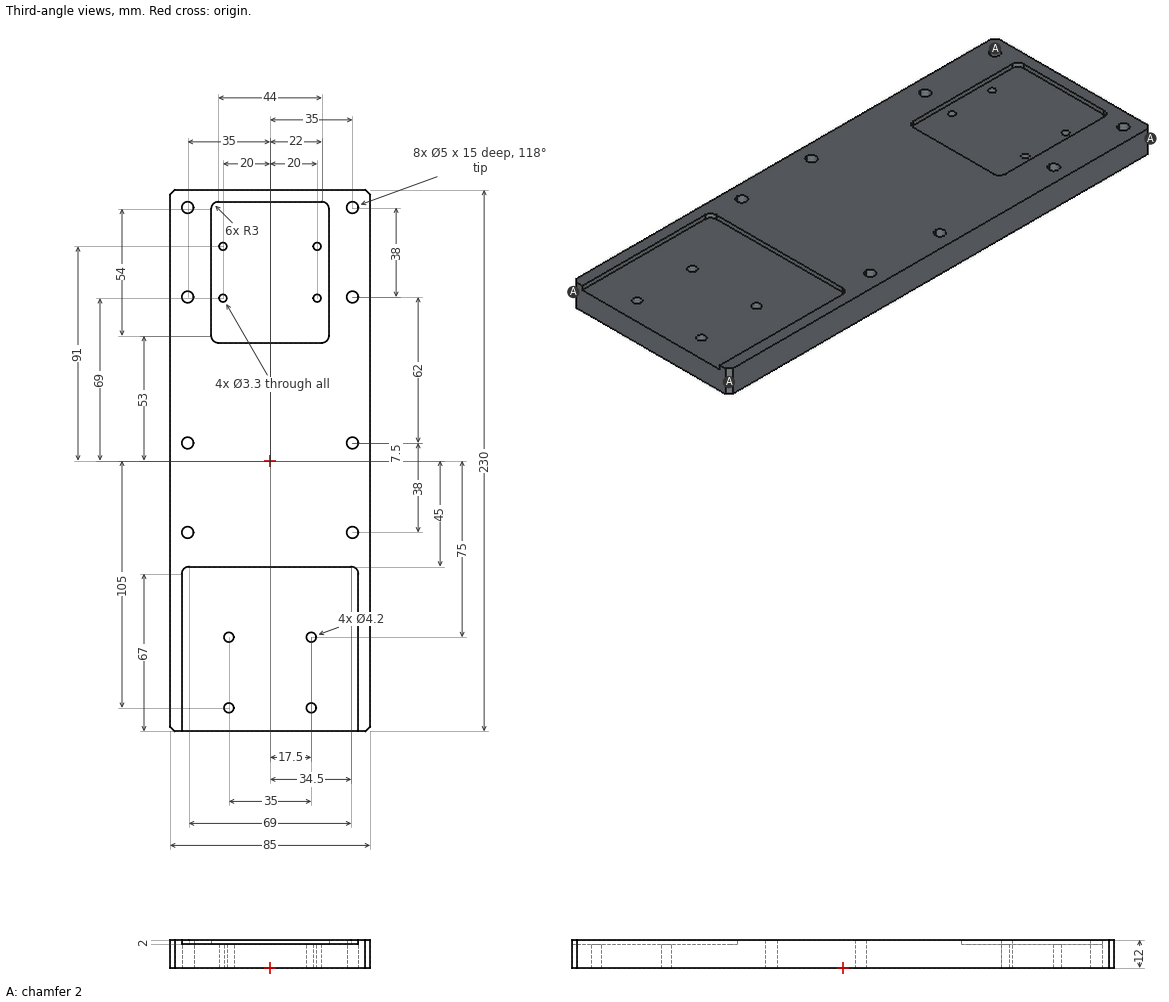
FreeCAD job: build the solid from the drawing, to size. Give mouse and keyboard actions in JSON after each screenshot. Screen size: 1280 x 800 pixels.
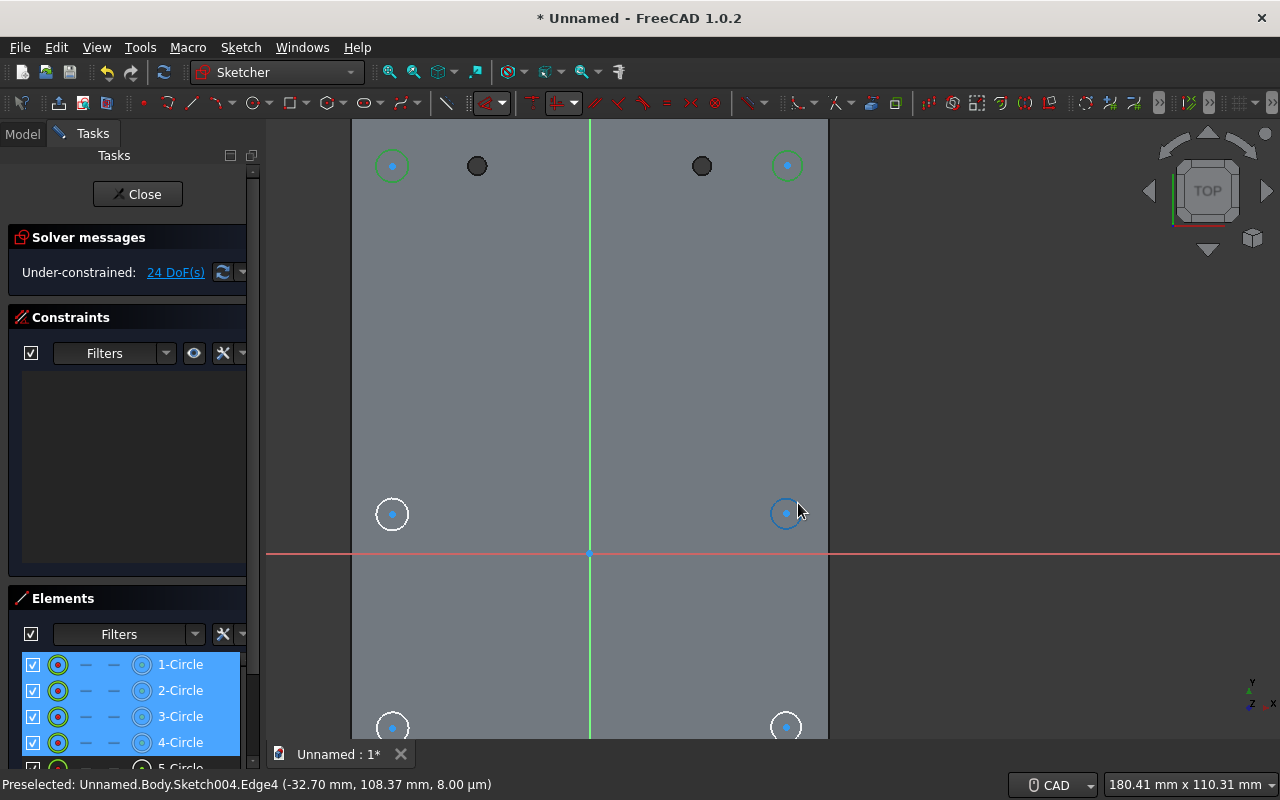
{"action": "left_click", "coordinate": [797, 503]}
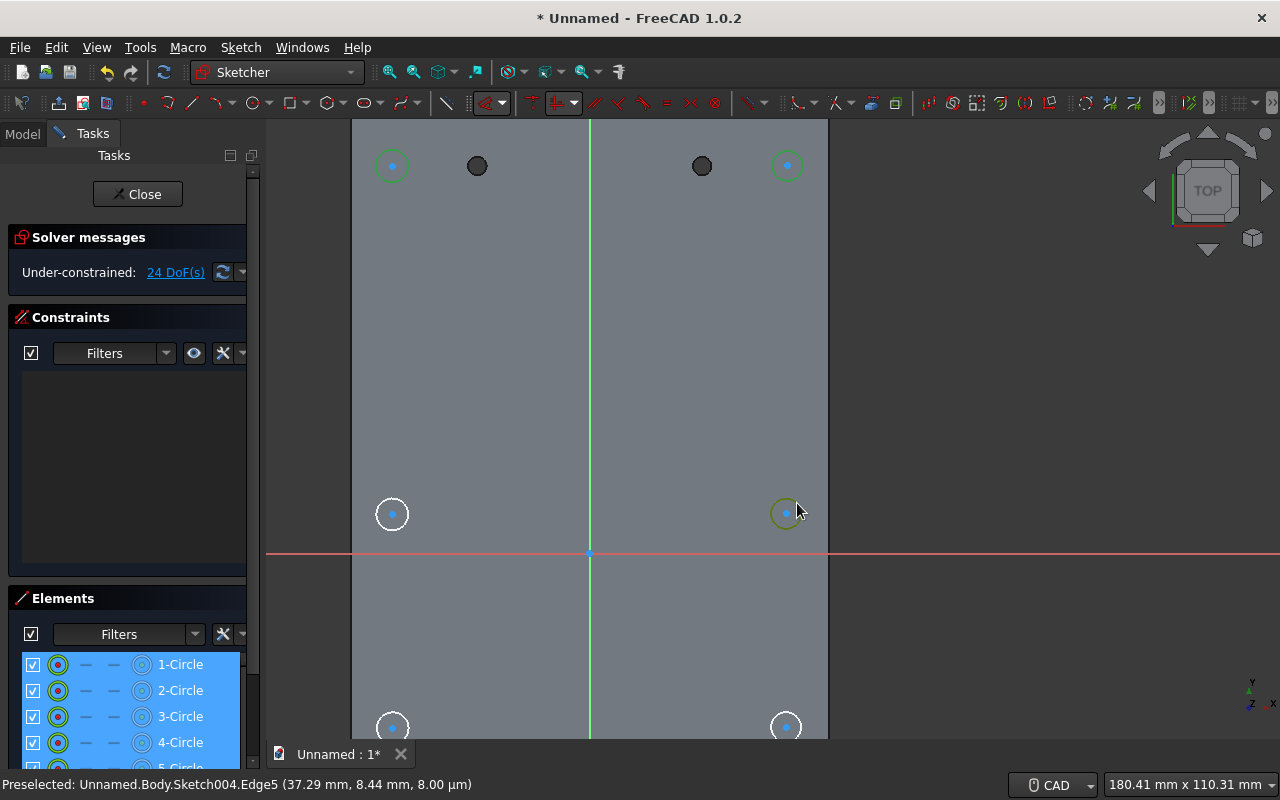
{"action": "scroll", "coordinate": [798, 504], "scroll_direction": "down", "scroll_amount": 4}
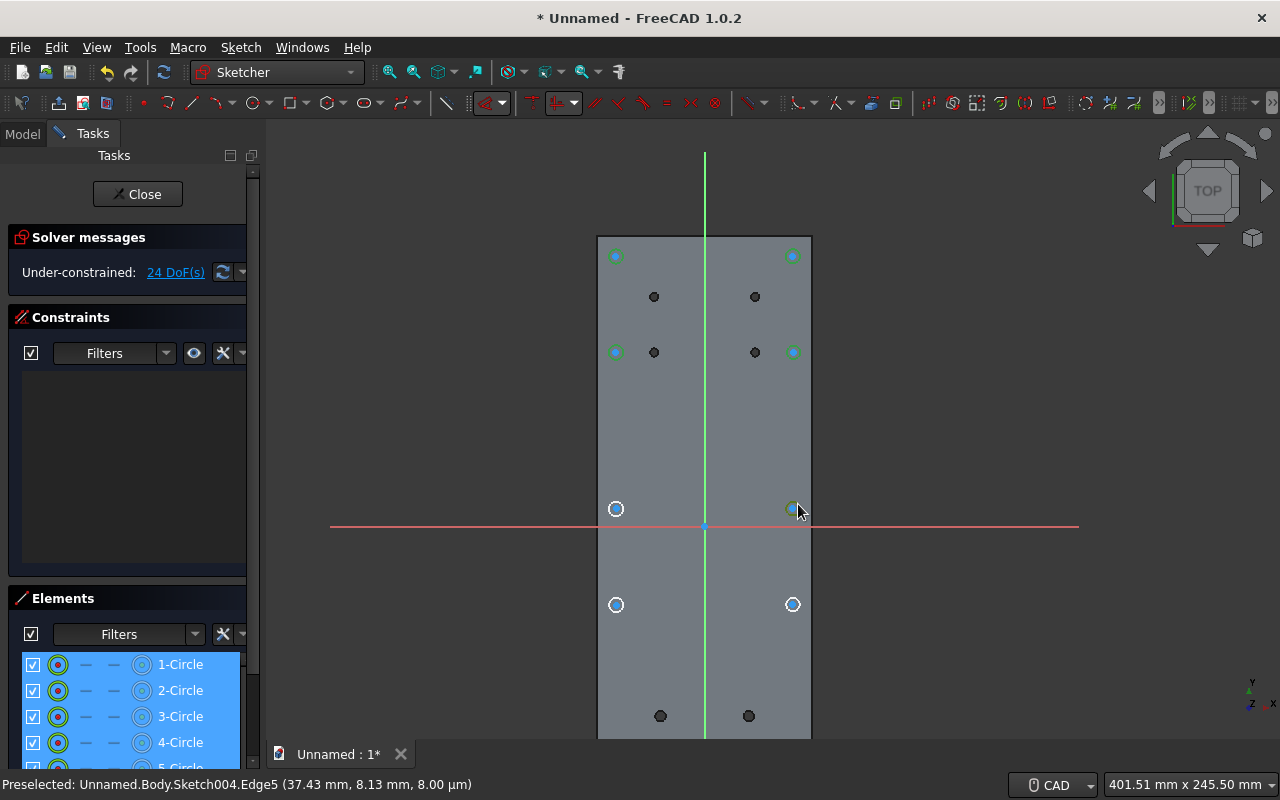
{"action": "scroll", "coordinate": [798, 600], "scroll_direction": "up", "scroll_amount": 4}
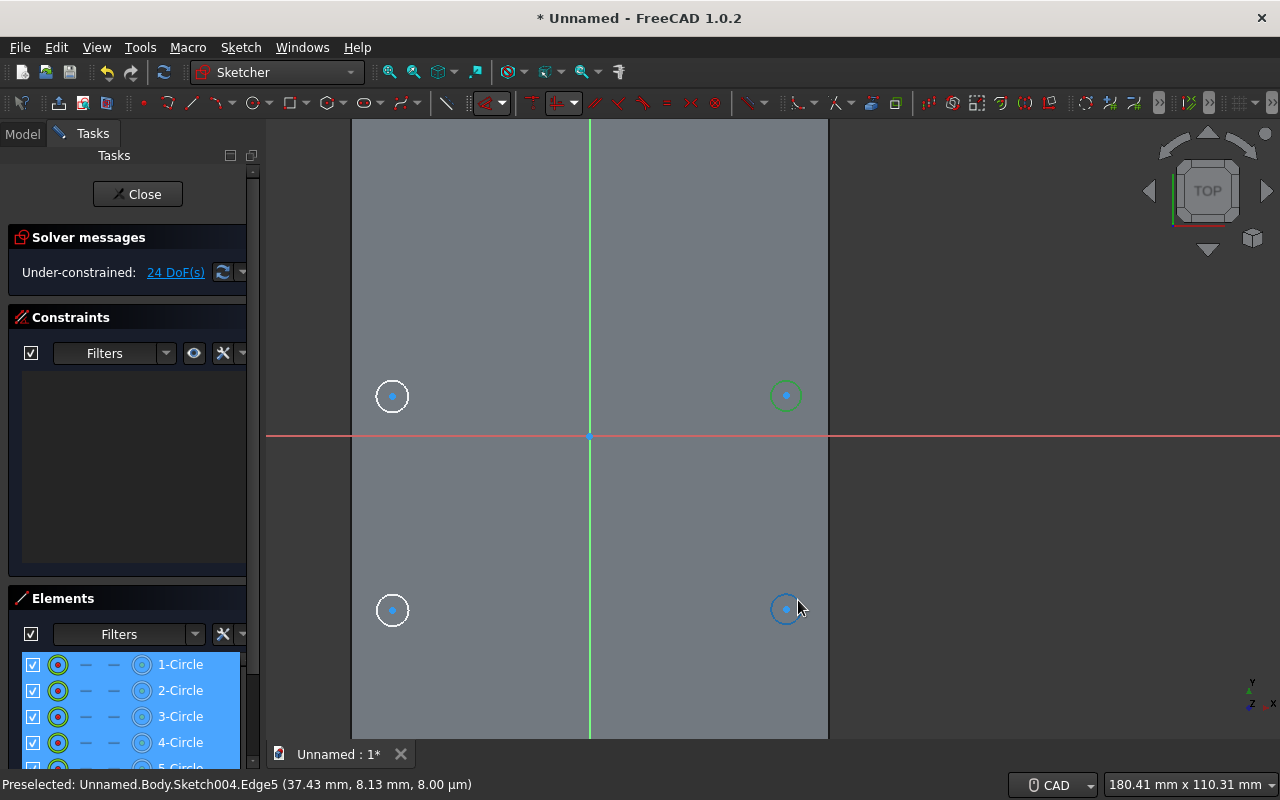
{"action": "left_click", "coordinate": [797, 599]}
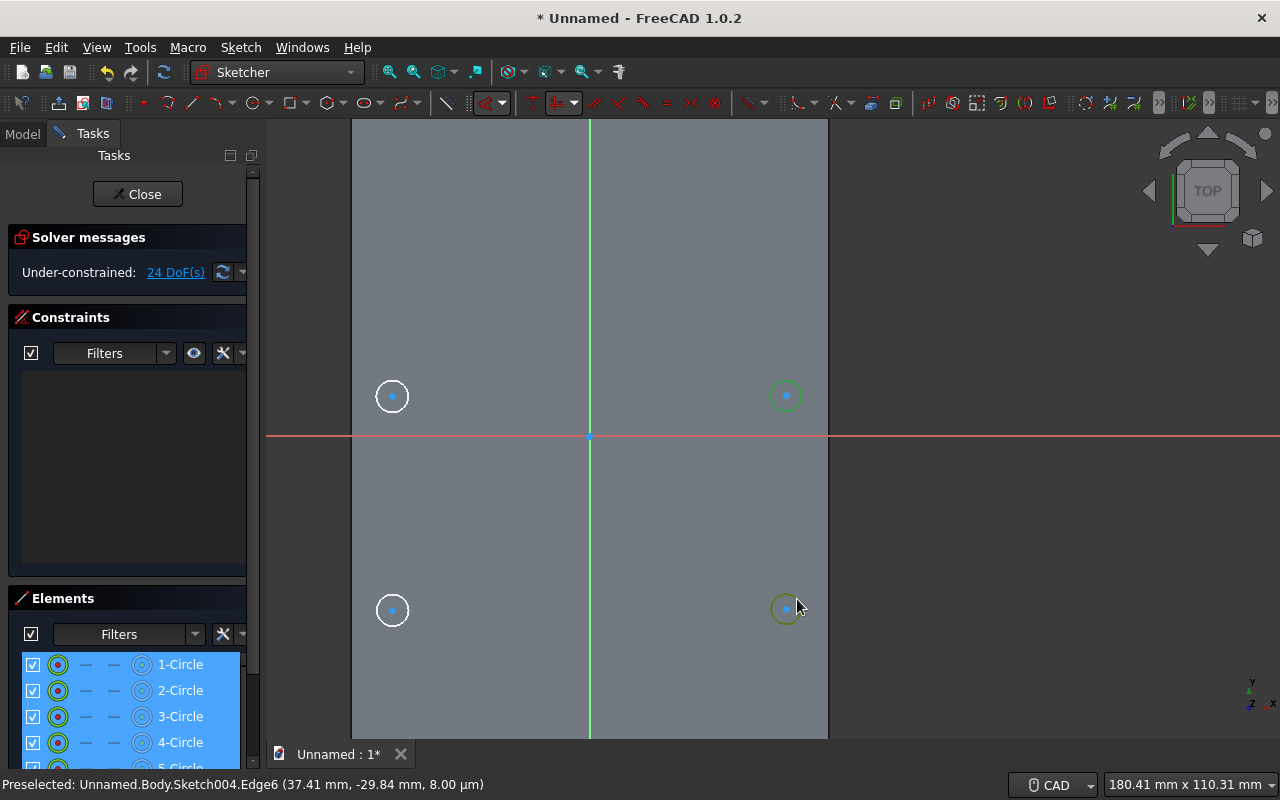
{"action": "left_click", "coordinate": [404, 599]}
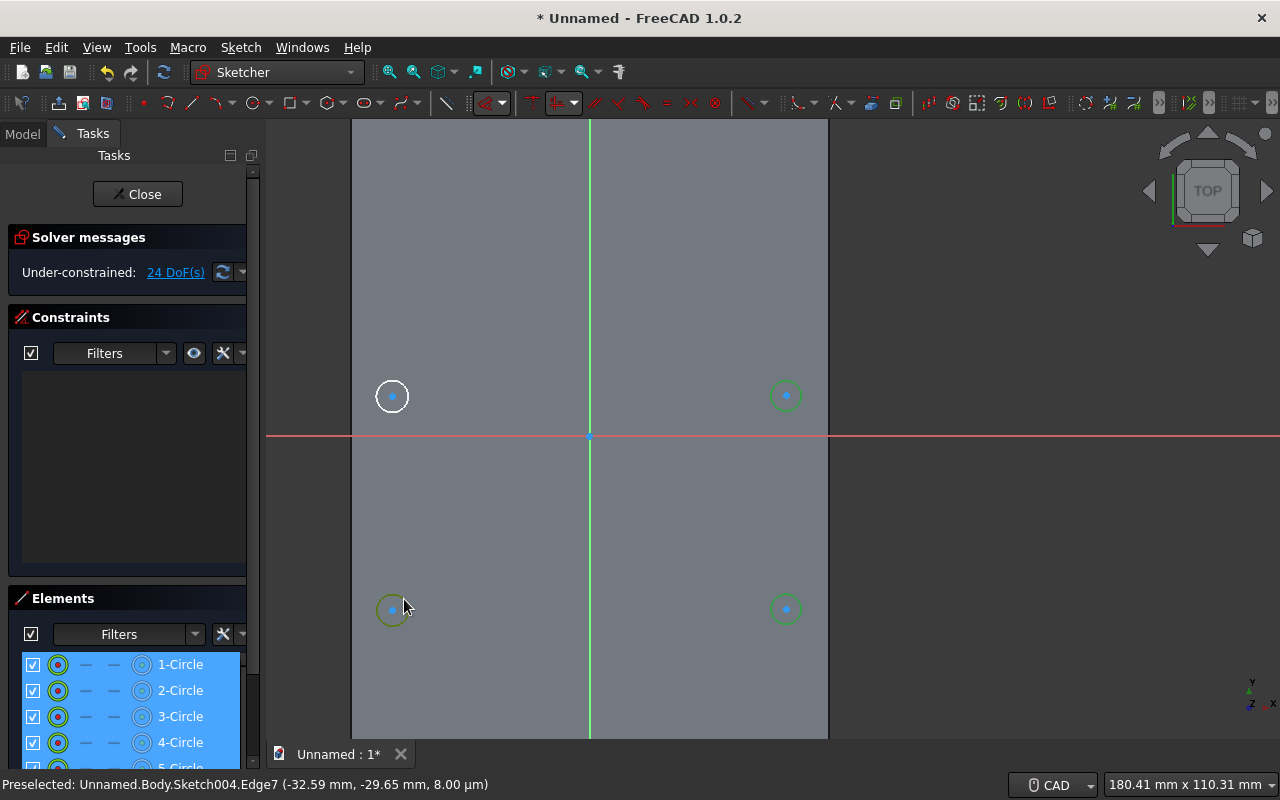
{"action": "left_click", "coordinate": [404, 385]}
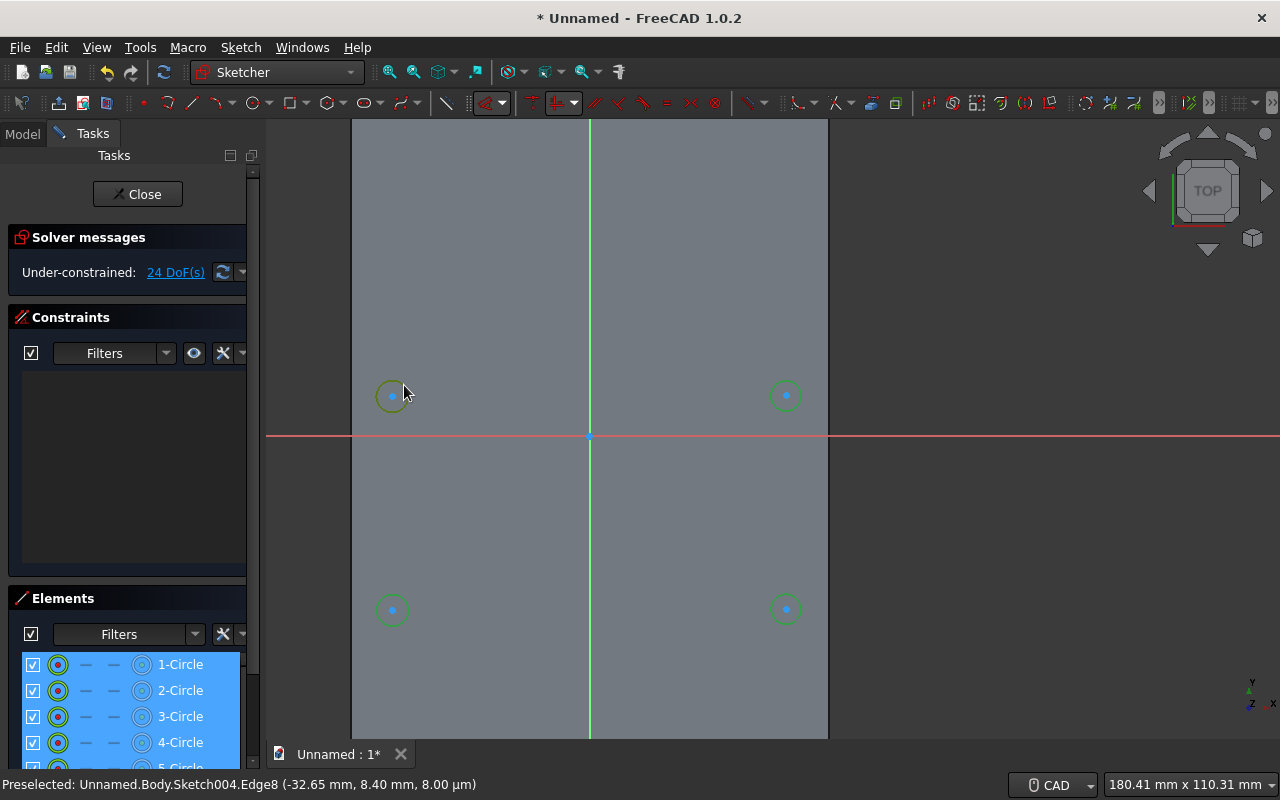
{"action": "key", "text": "e"}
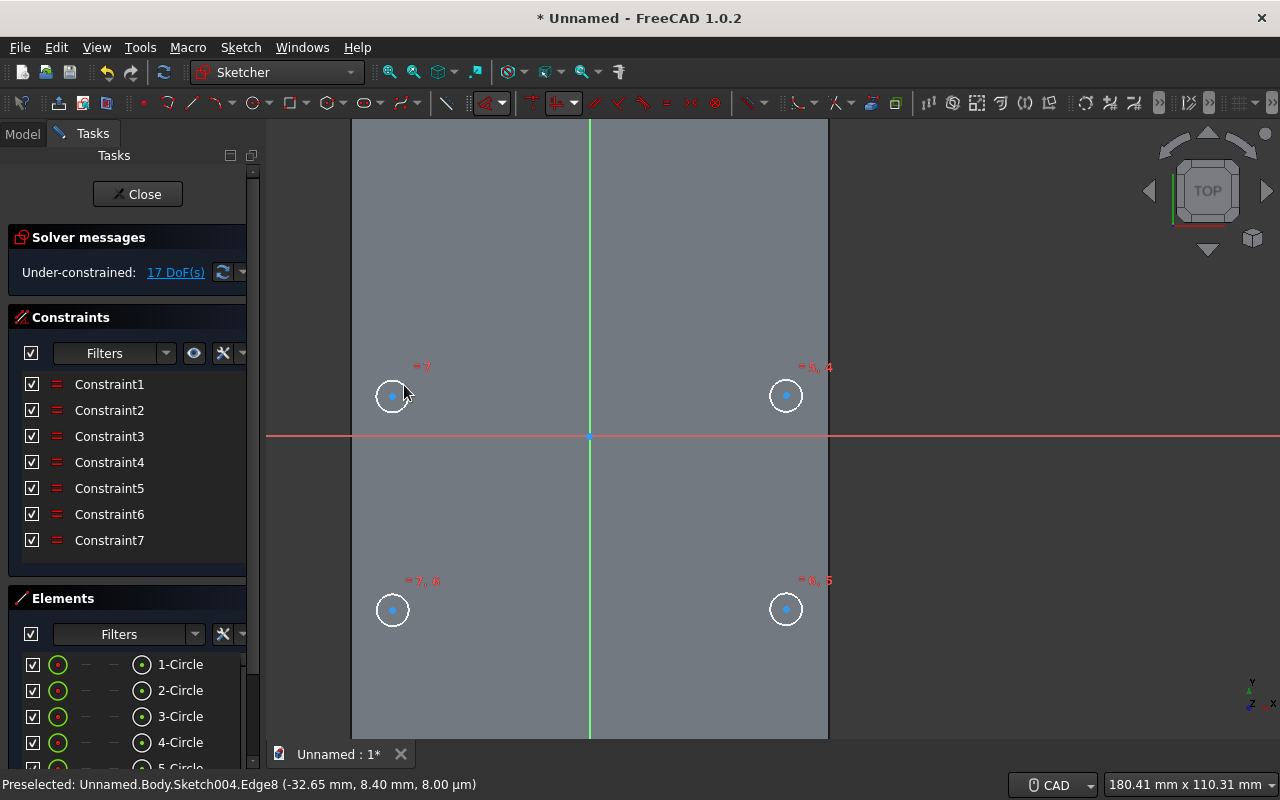
{"action": "scroll", "coordinate": [798, 600], "scroll_direction": "down", "scroll_amount": 4}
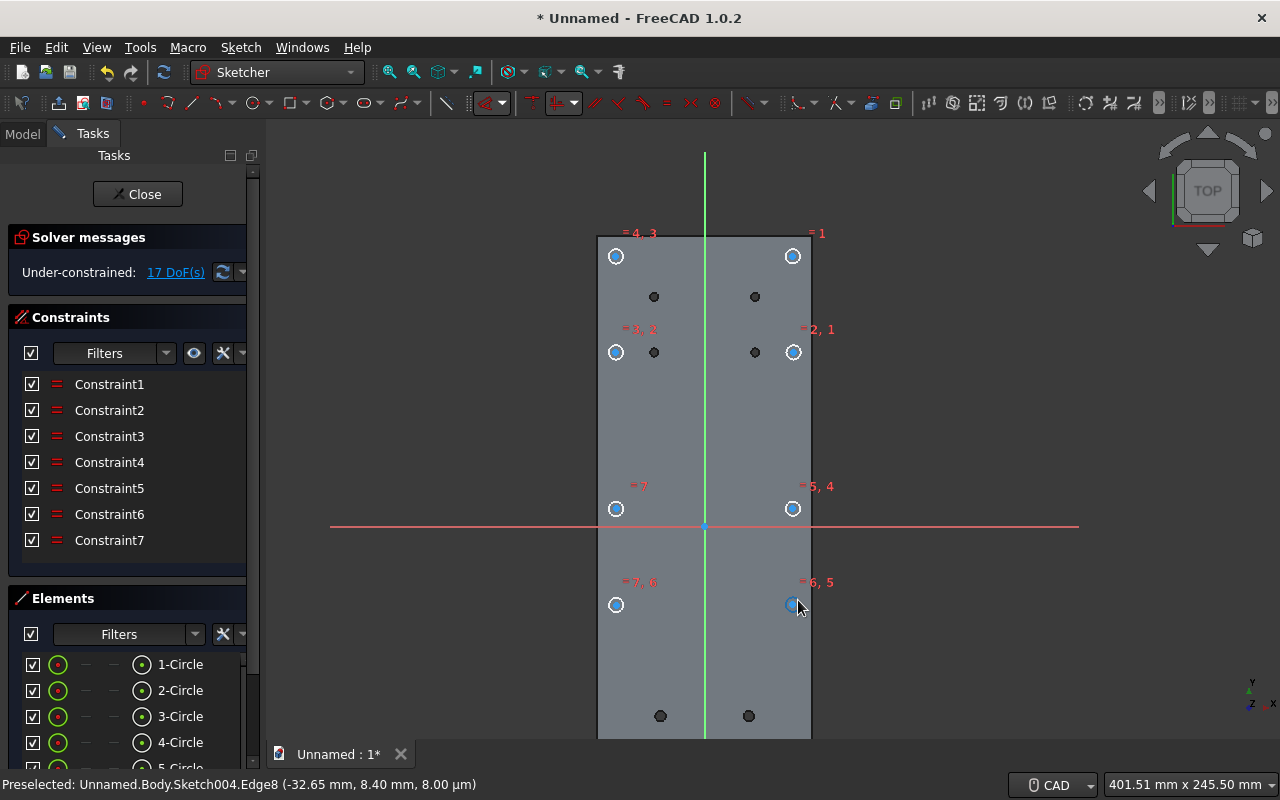
{"action": "left_click", "coordinate": [793, 256]}